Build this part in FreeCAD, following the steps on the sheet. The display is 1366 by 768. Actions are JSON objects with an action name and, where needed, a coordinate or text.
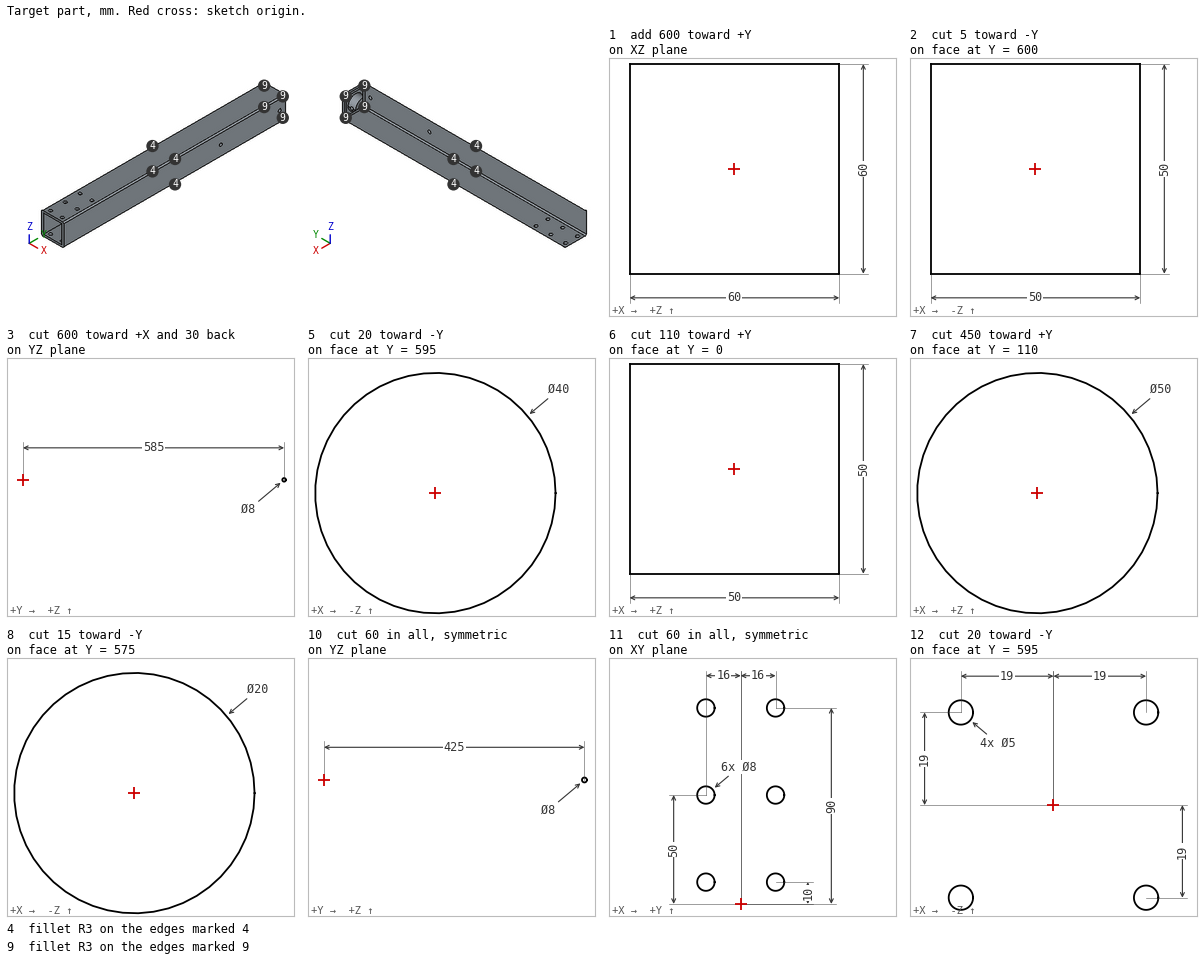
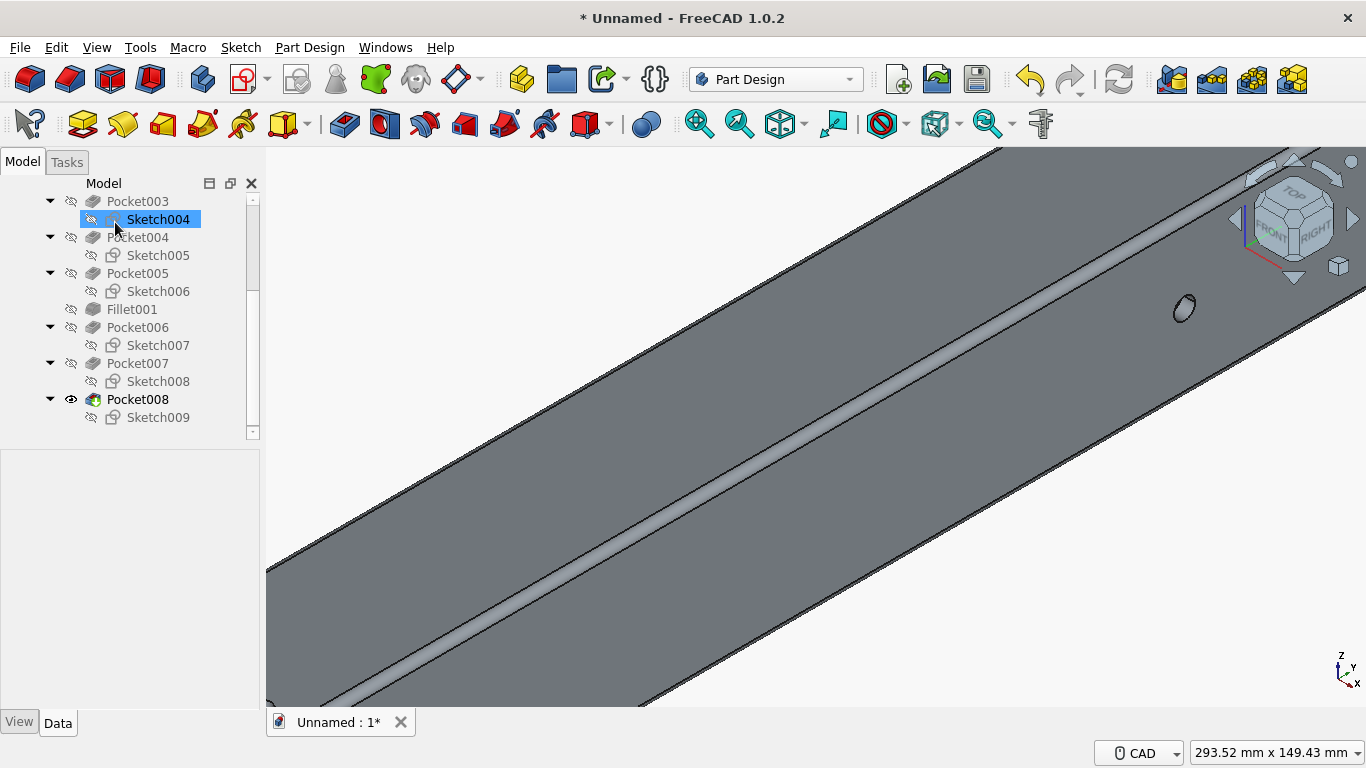
{"action": "key", "text": "v f"}